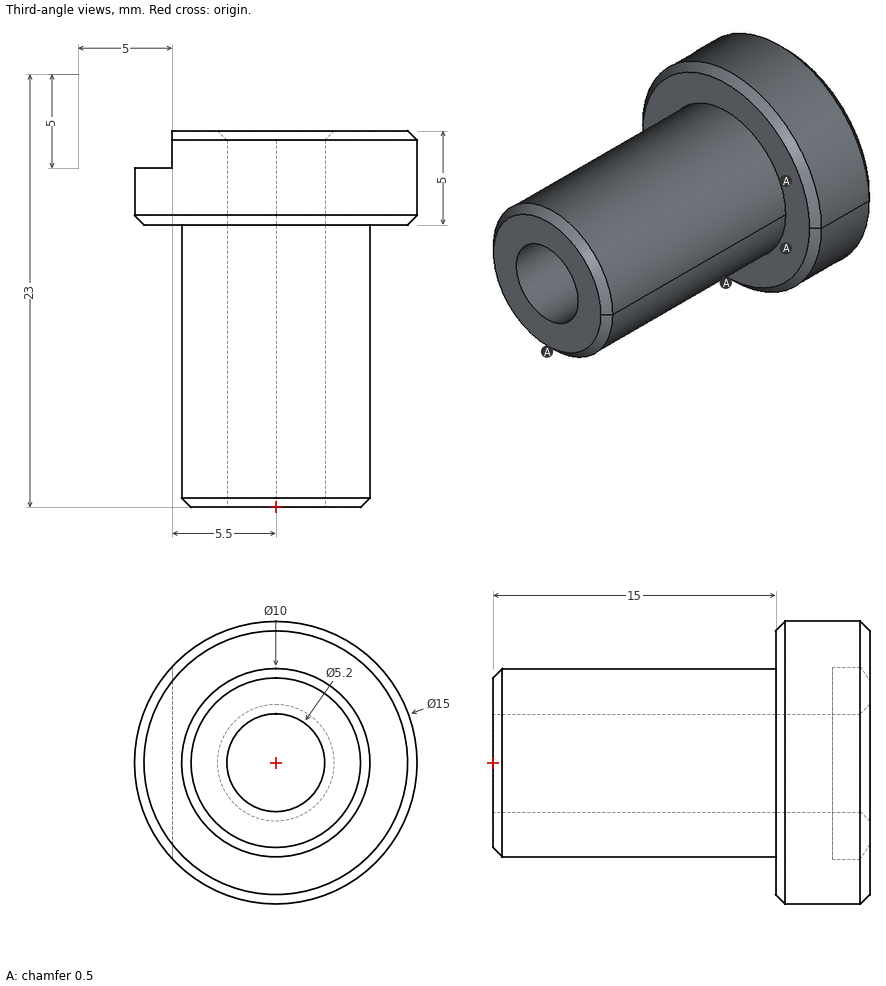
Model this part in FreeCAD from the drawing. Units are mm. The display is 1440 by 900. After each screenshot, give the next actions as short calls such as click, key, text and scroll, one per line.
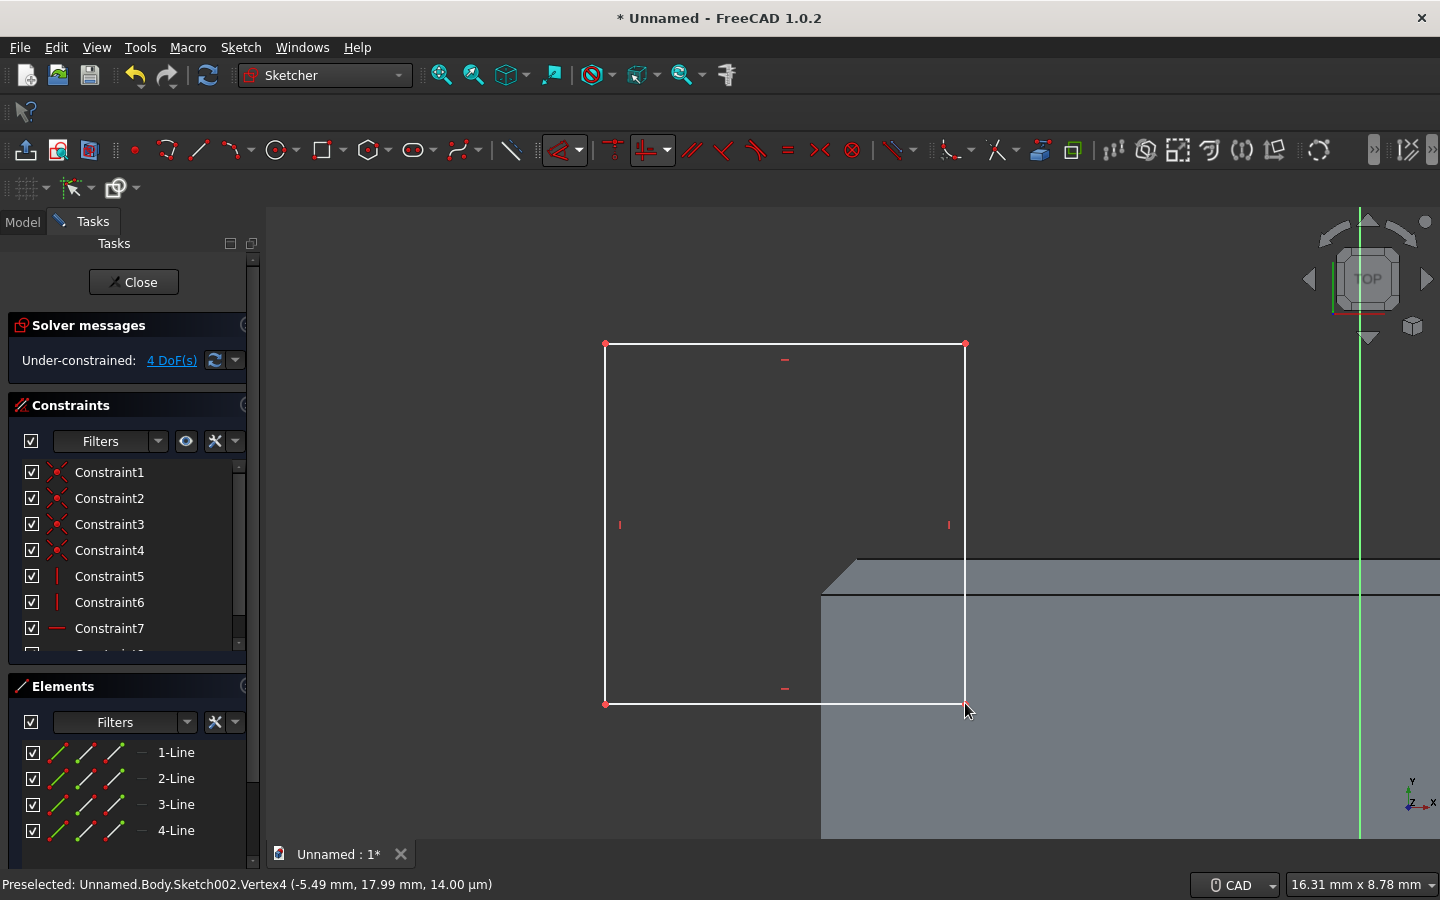
click(605, 452)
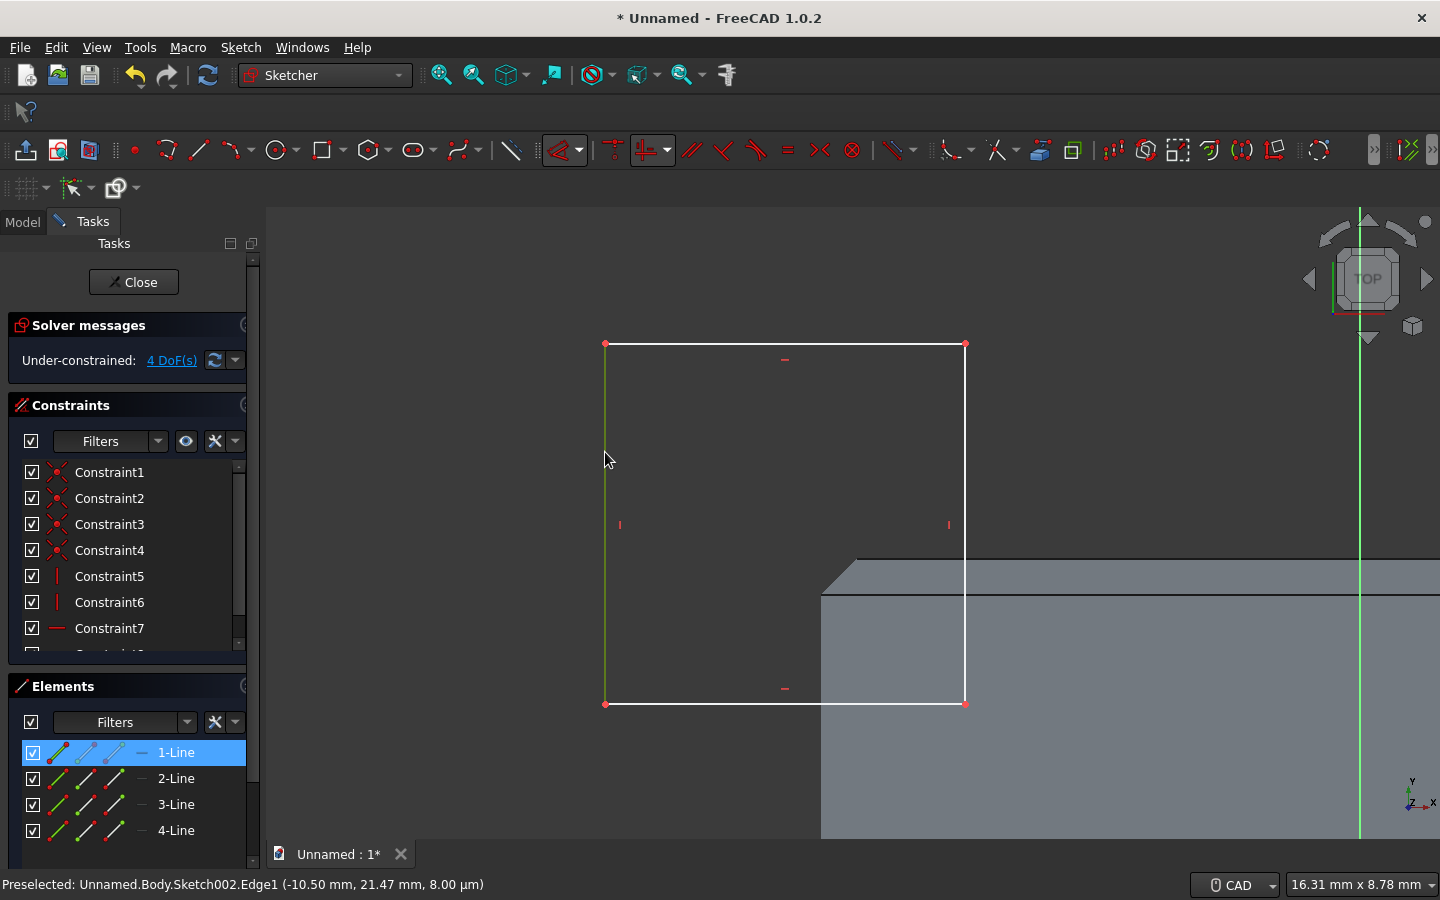
click(582, 150)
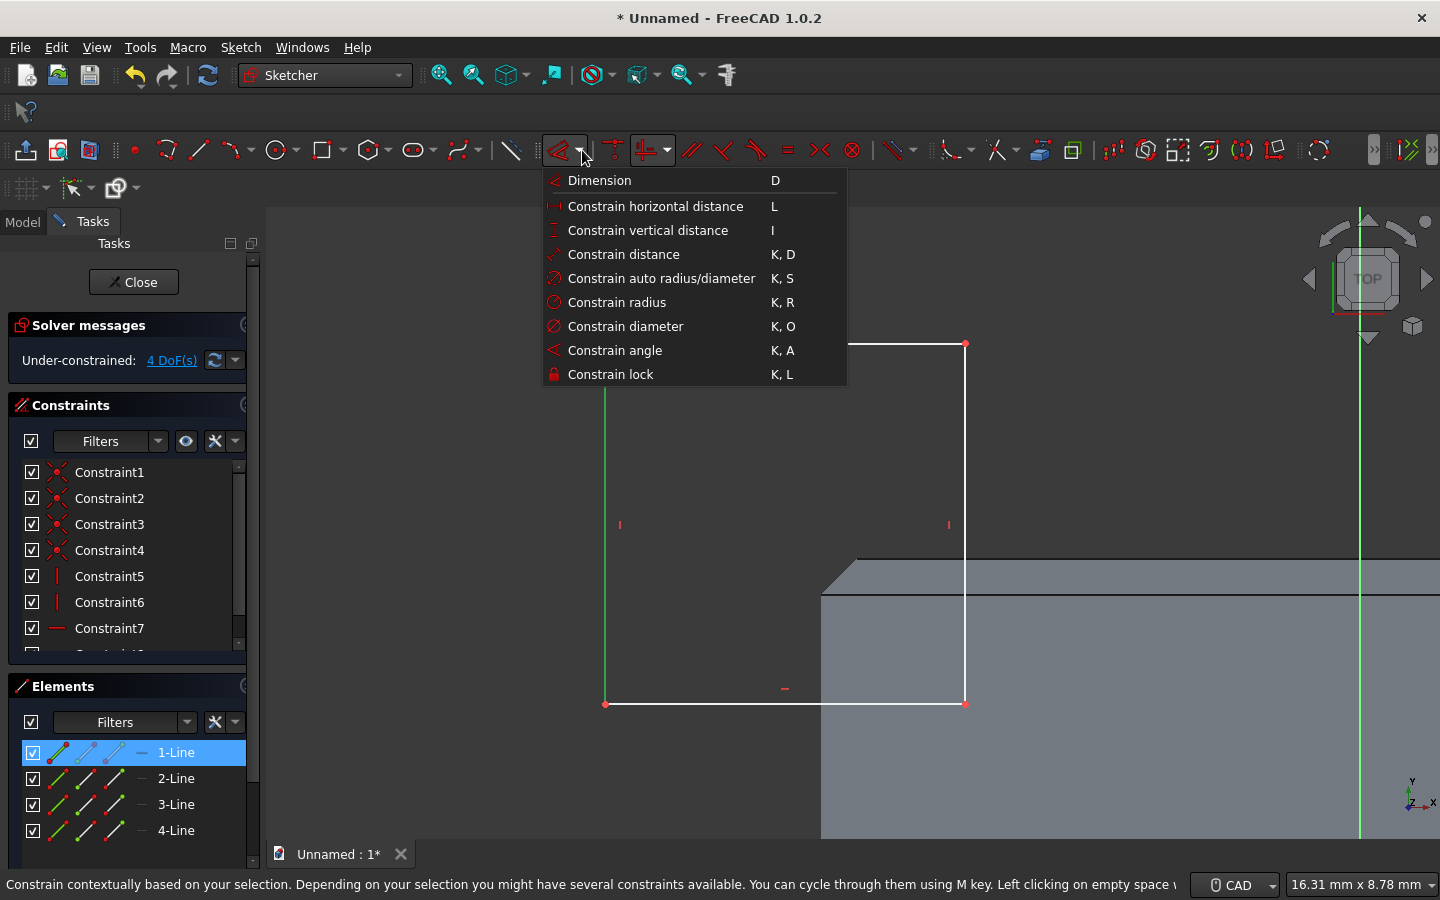
click(695, 230)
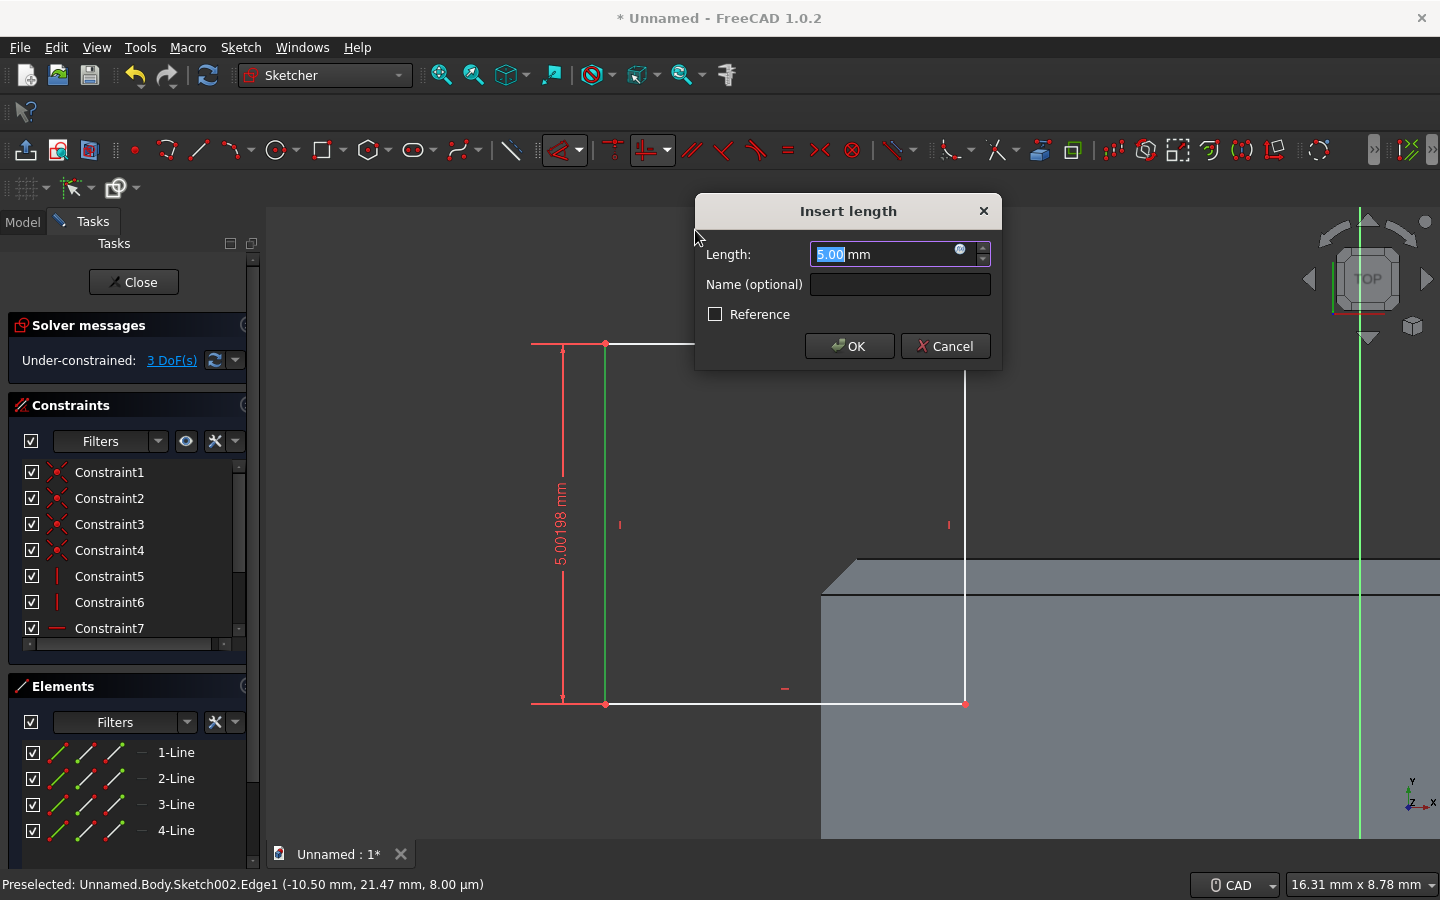
text(5)
key(Return)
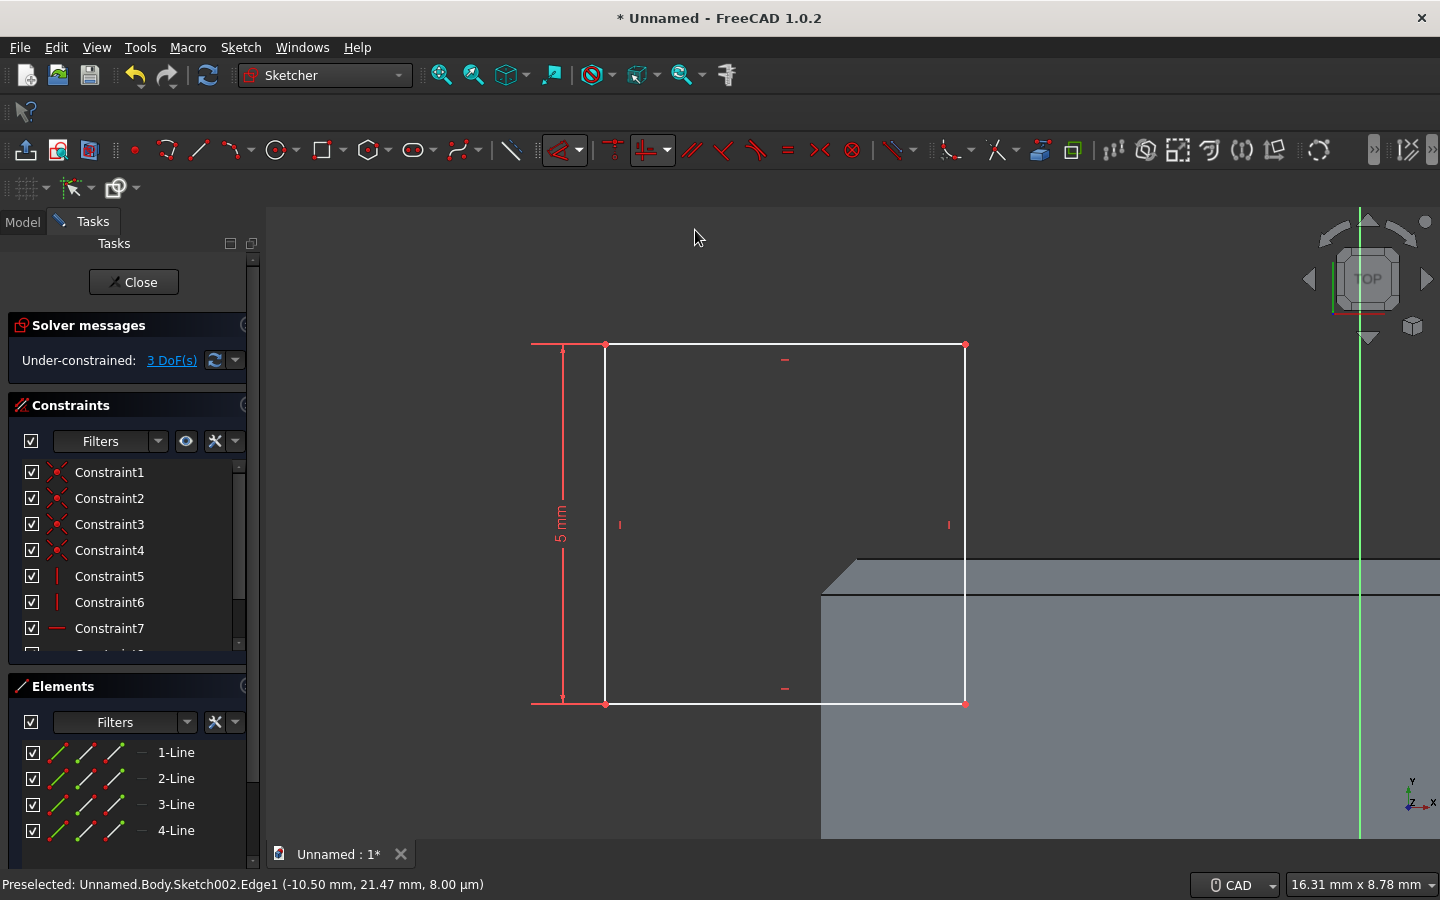
click(713, 704)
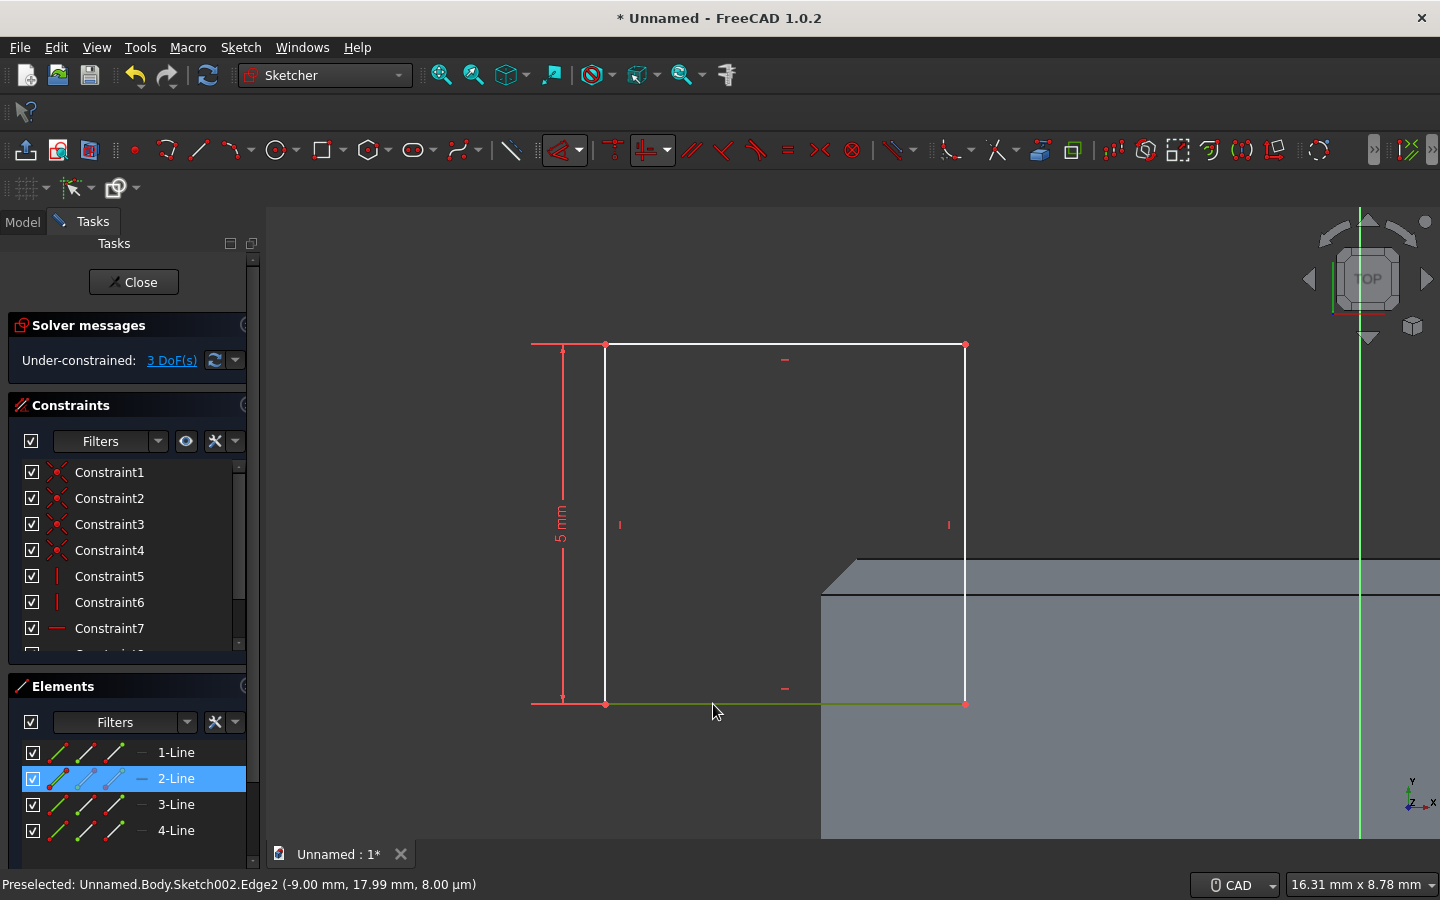
key(l)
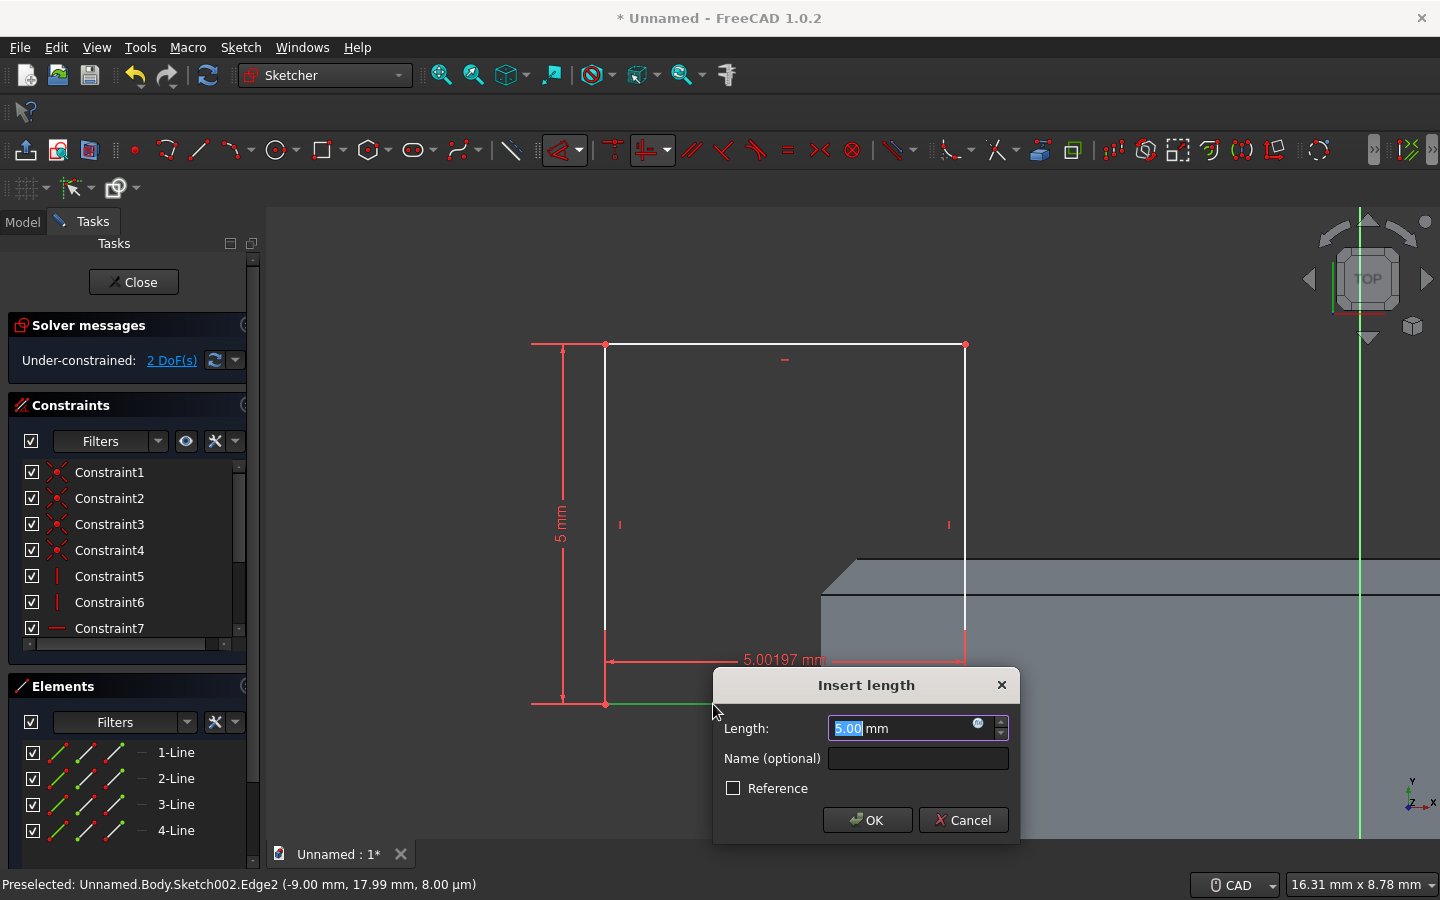
text(5)
key(Return)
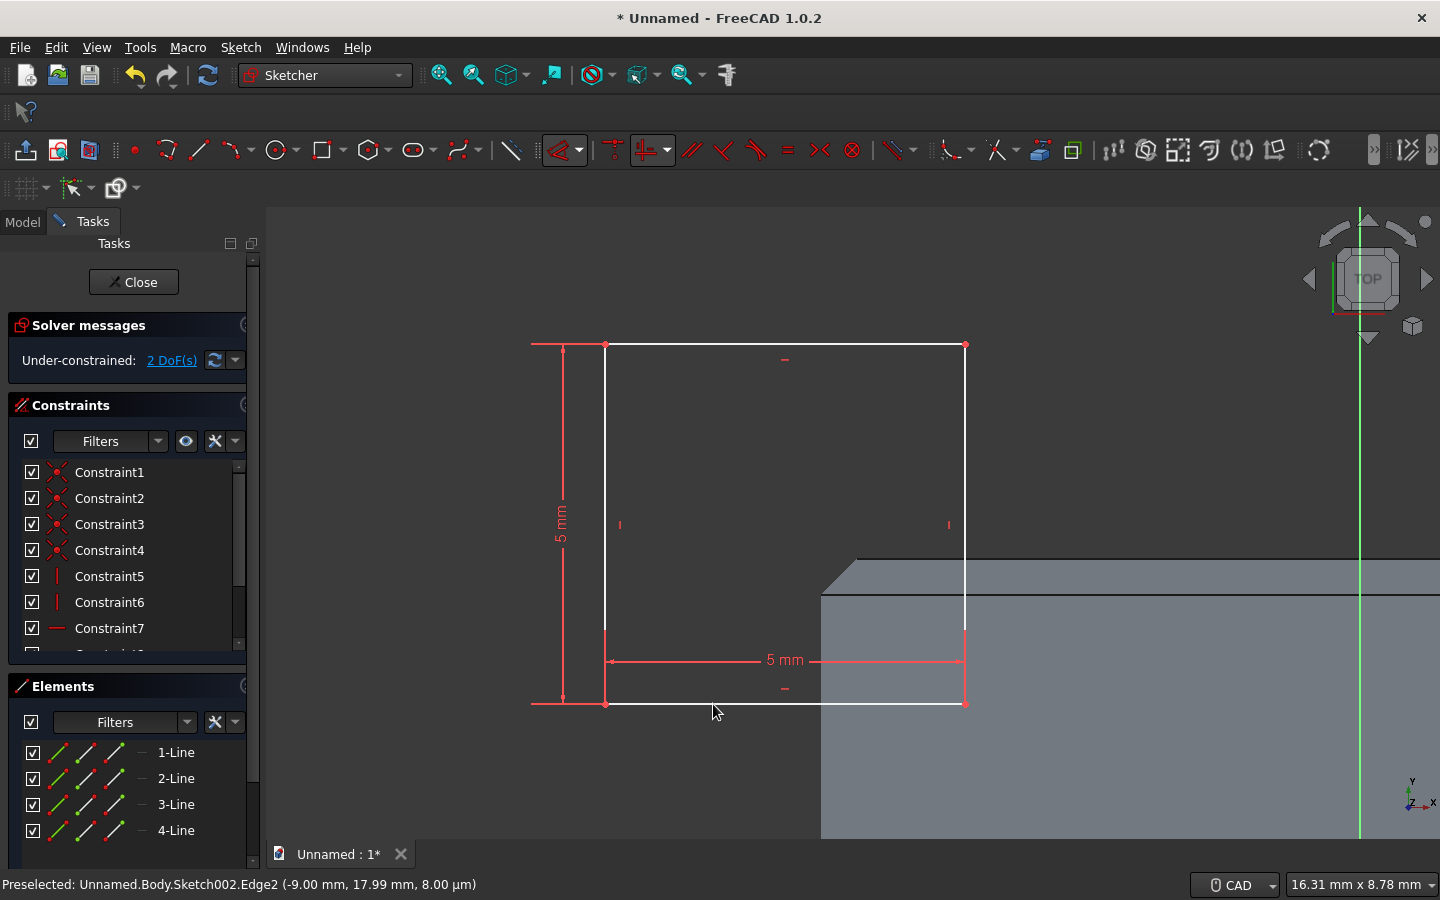
click(605, 344)